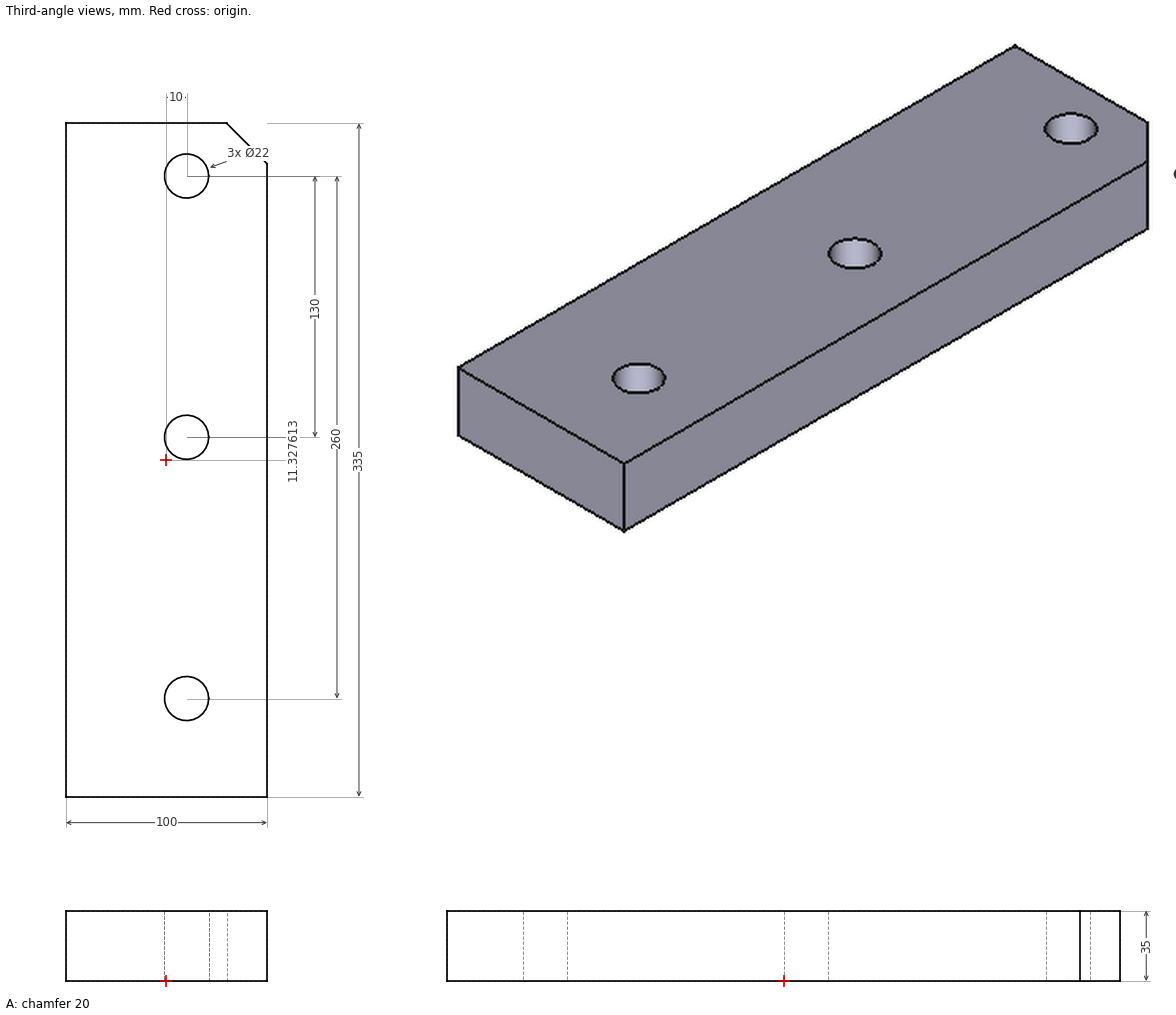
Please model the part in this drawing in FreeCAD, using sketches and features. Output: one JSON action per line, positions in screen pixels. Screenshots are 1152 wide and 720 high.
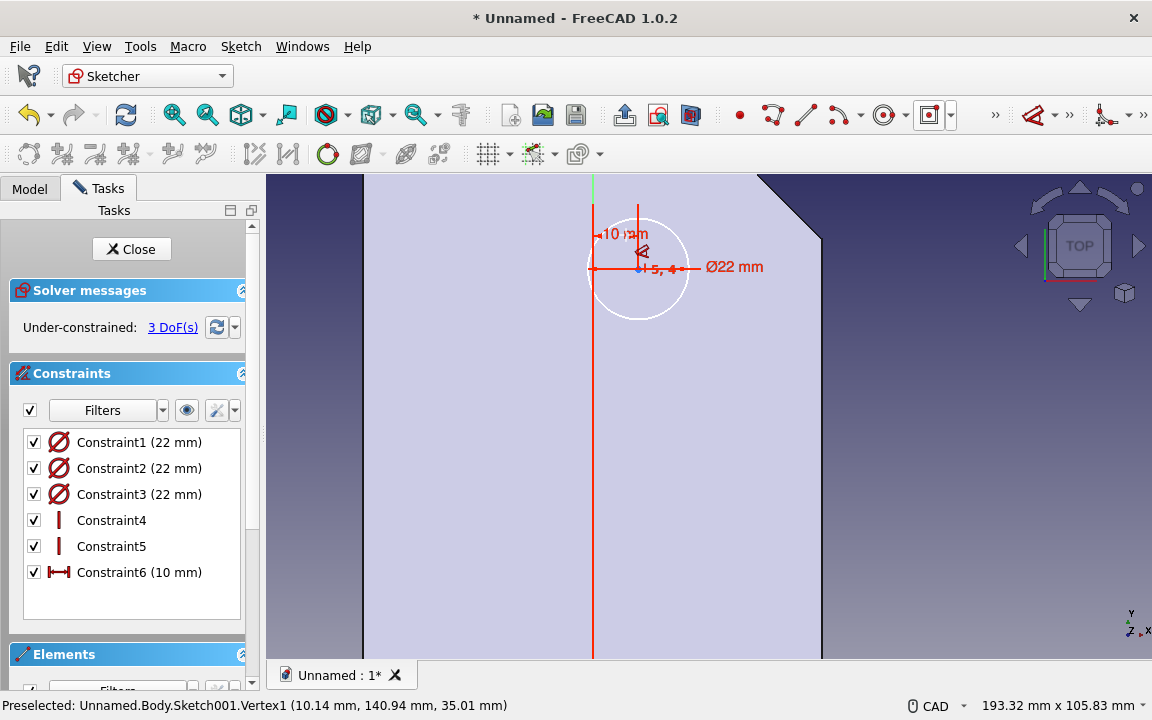
{"action": "scroll", "coordinate": [641, 270], "scroll_direction": "down", "scroll_amount": 7}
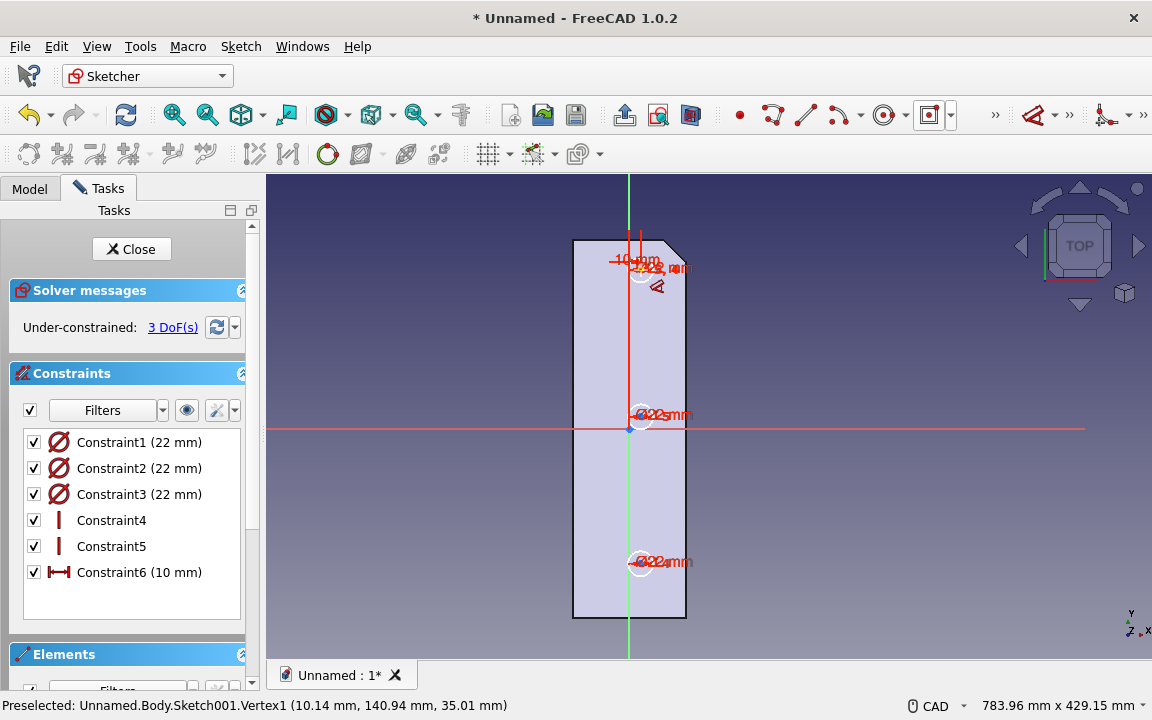
{"action": "left_click", "coordinate": [641, 270]}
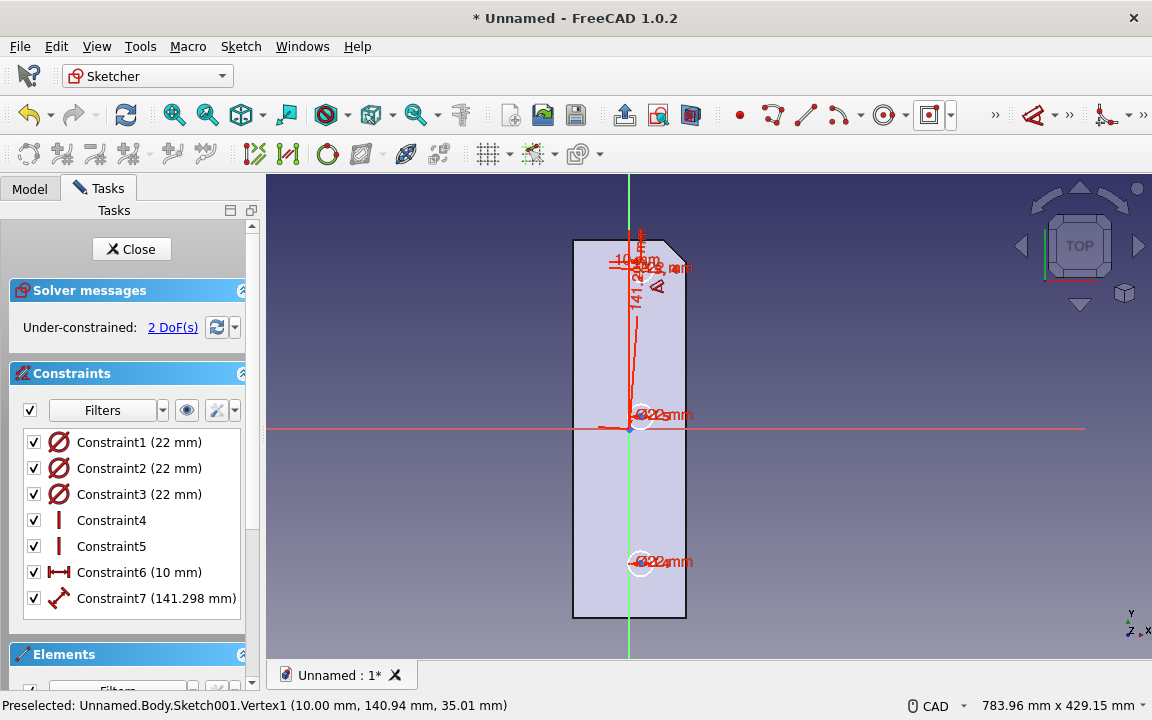
{"action": "left_click", "coordinate": [641, 564]}
{"action": "left_click", "coordinate": [675, 349]}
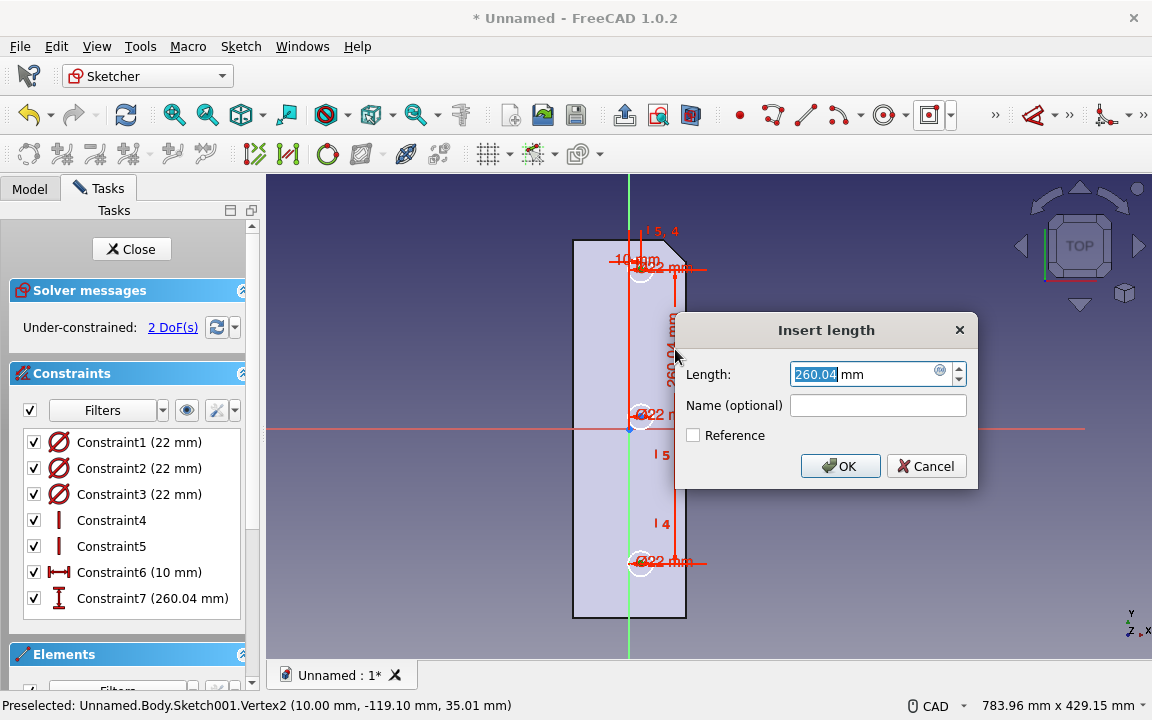
{"action": "type", "text": "260"}
{"action": "key", "text": "Return"}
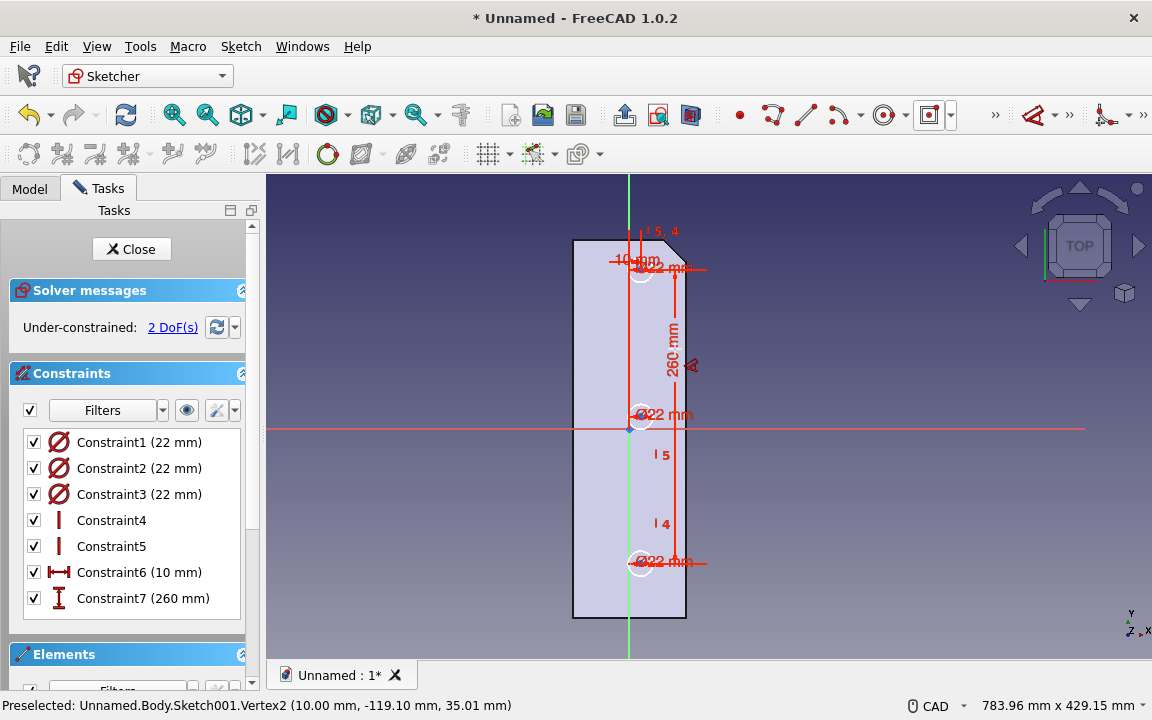
{"action": "left_click", "coordinate": [641, 270]}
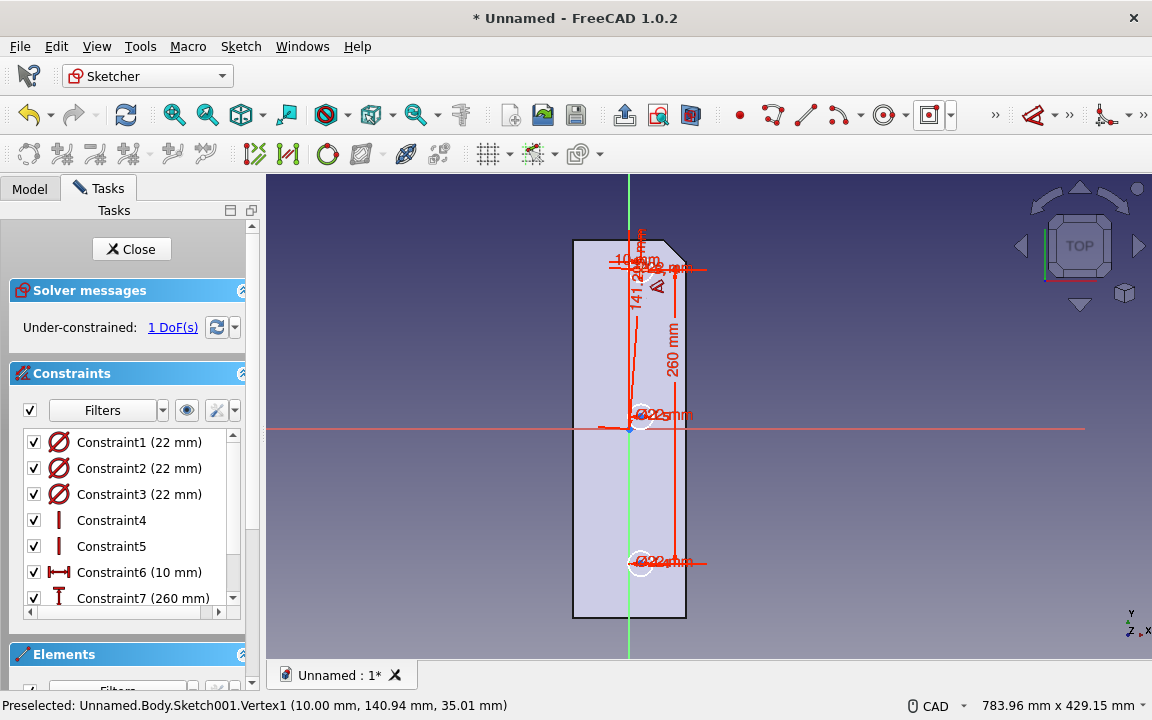
{"action": "left_click", "coordinate": [641, 417]}
{"action": "left_click", "coordinate": [675, 310]}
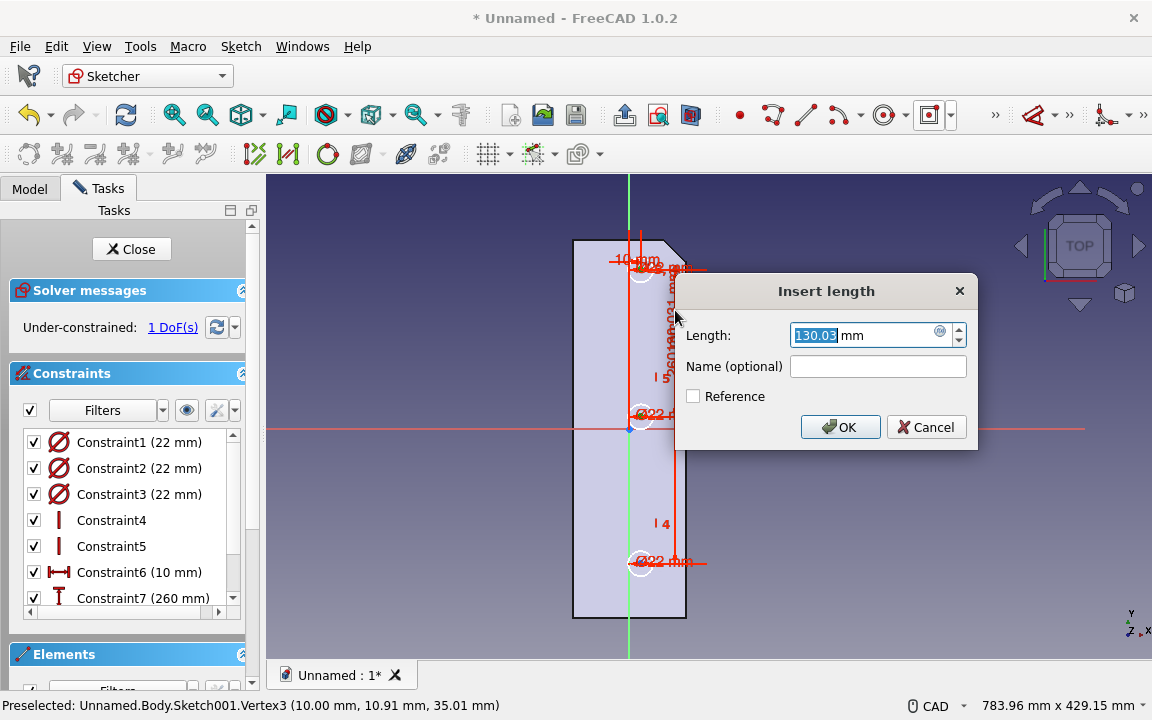
{"action": "type", "text": "130"}
{"action": "key", "text": "Return"}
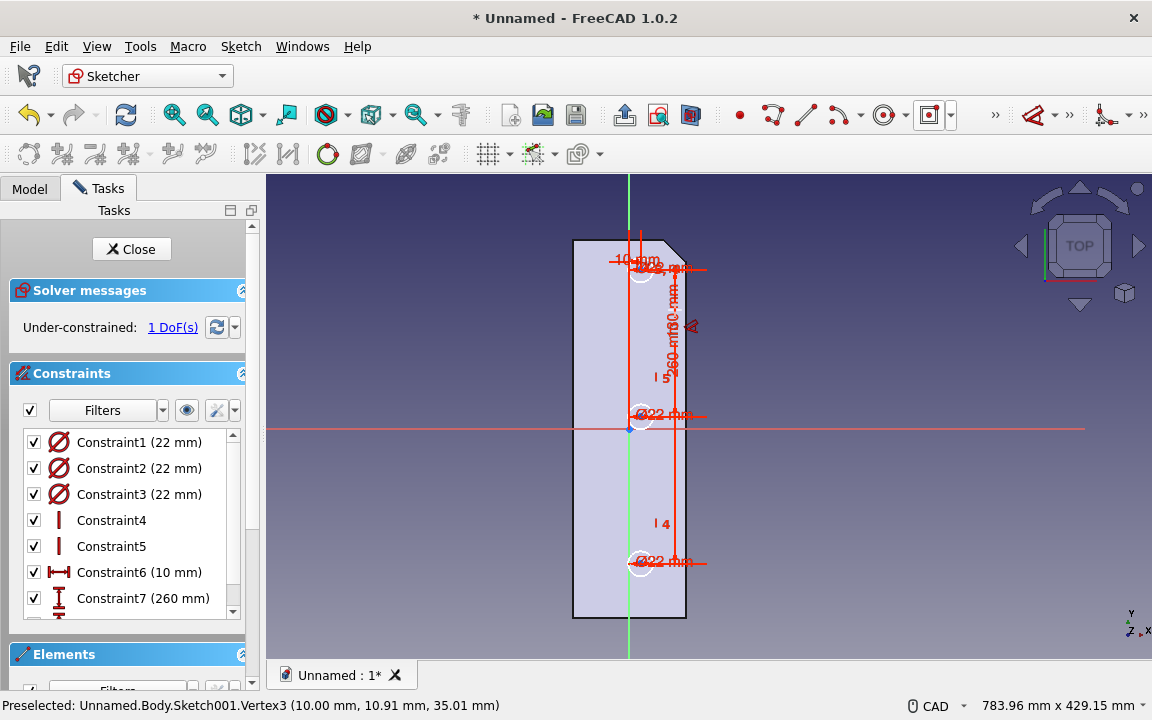
{"action": "scroll", "coordinate": [641, 417], "scroll_direction": "up", "scroll_amount": 6}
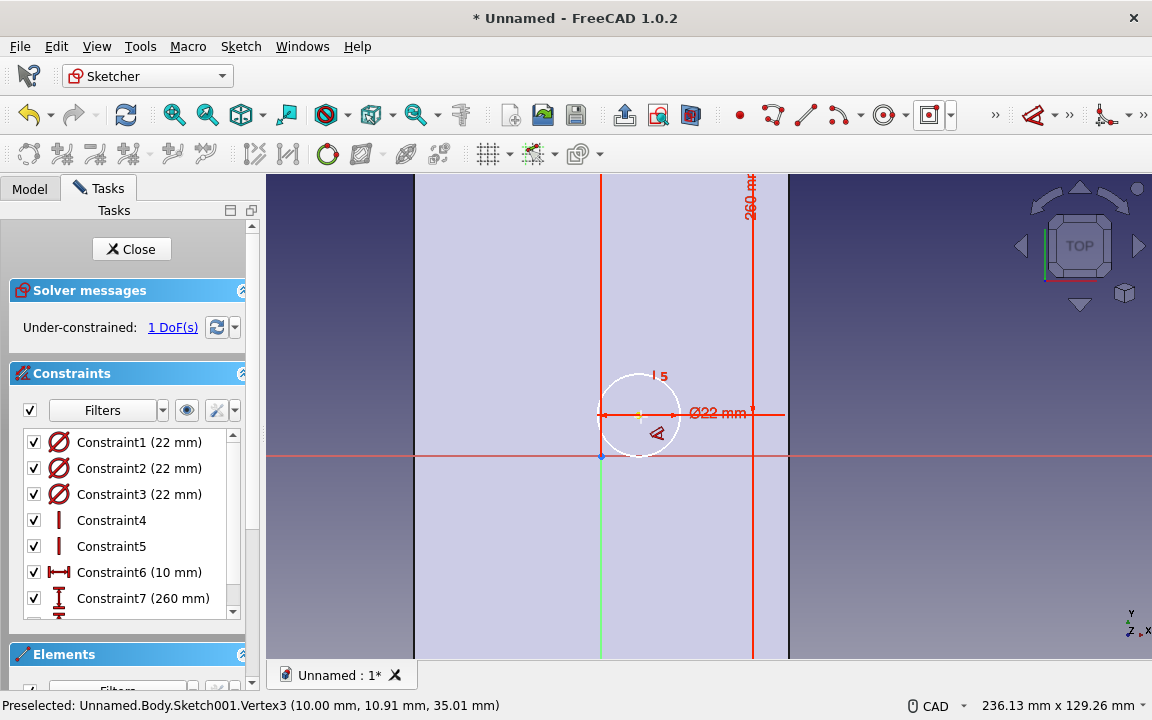
{"action": "left_click", "coordinate": [639, 415]}
{"action": "left_click", "coordinate": [567, 436]}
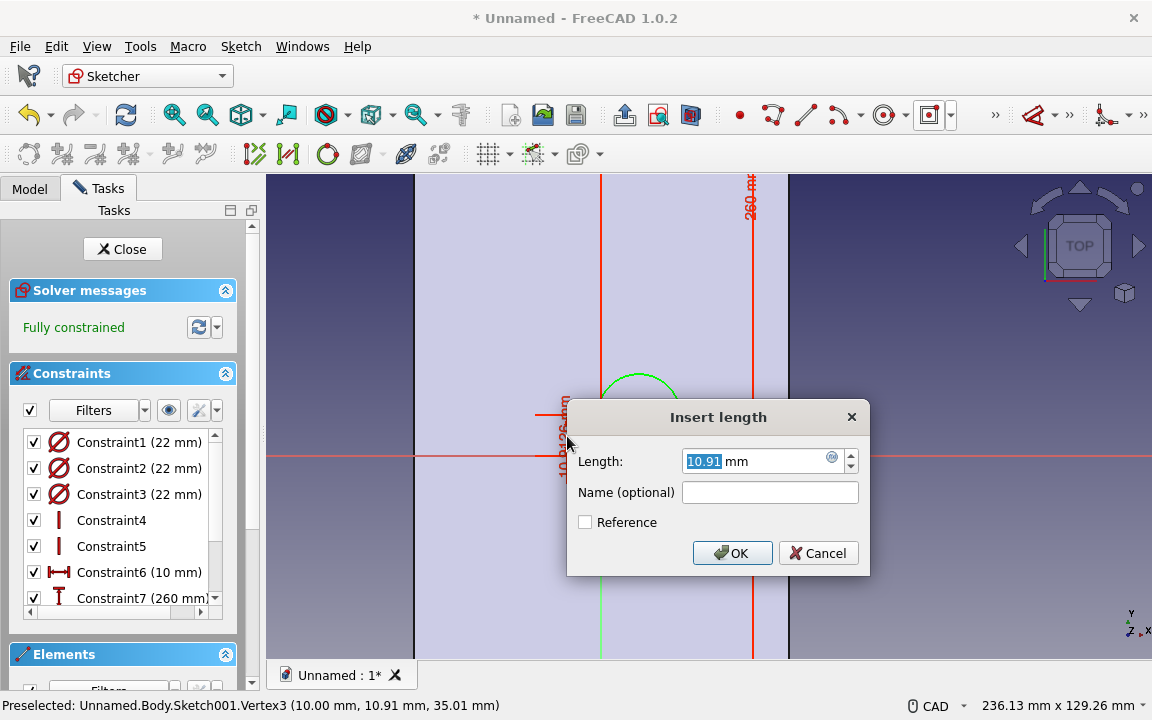
{"action": "type", "text": "11.327613"}
{"action": "key", "text": "Return"}
{"action": "key", "text": "Escape"}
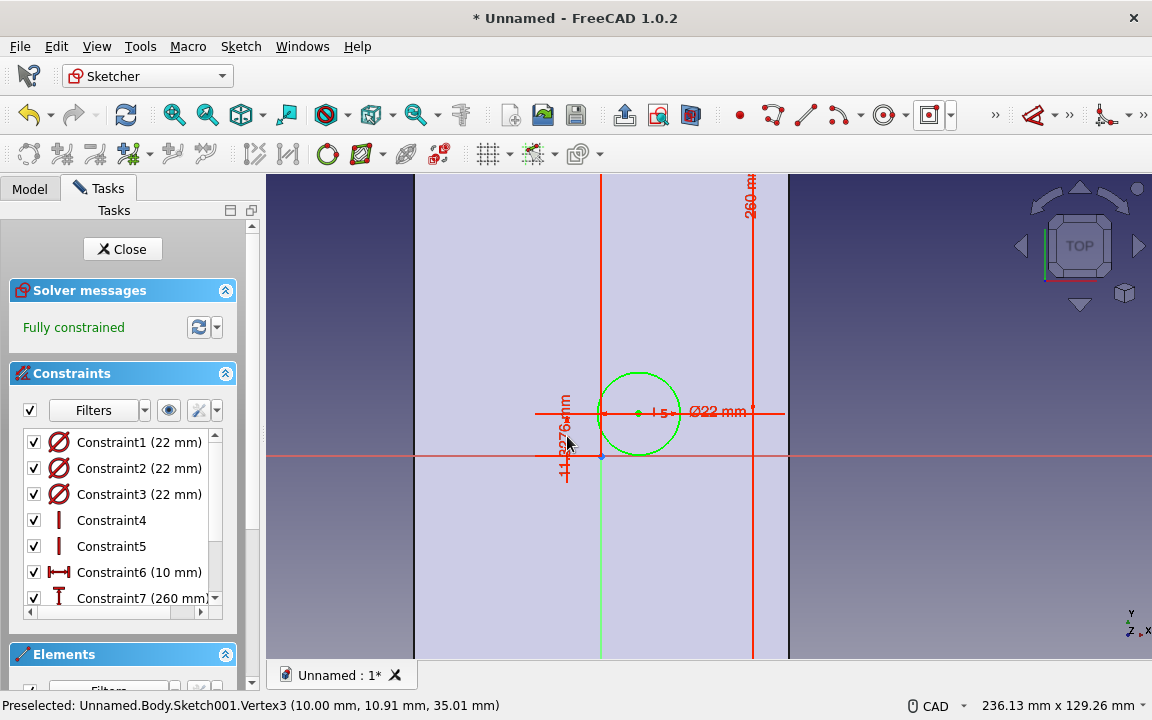
{"action": "left_click", "coordinate": [123, 249]}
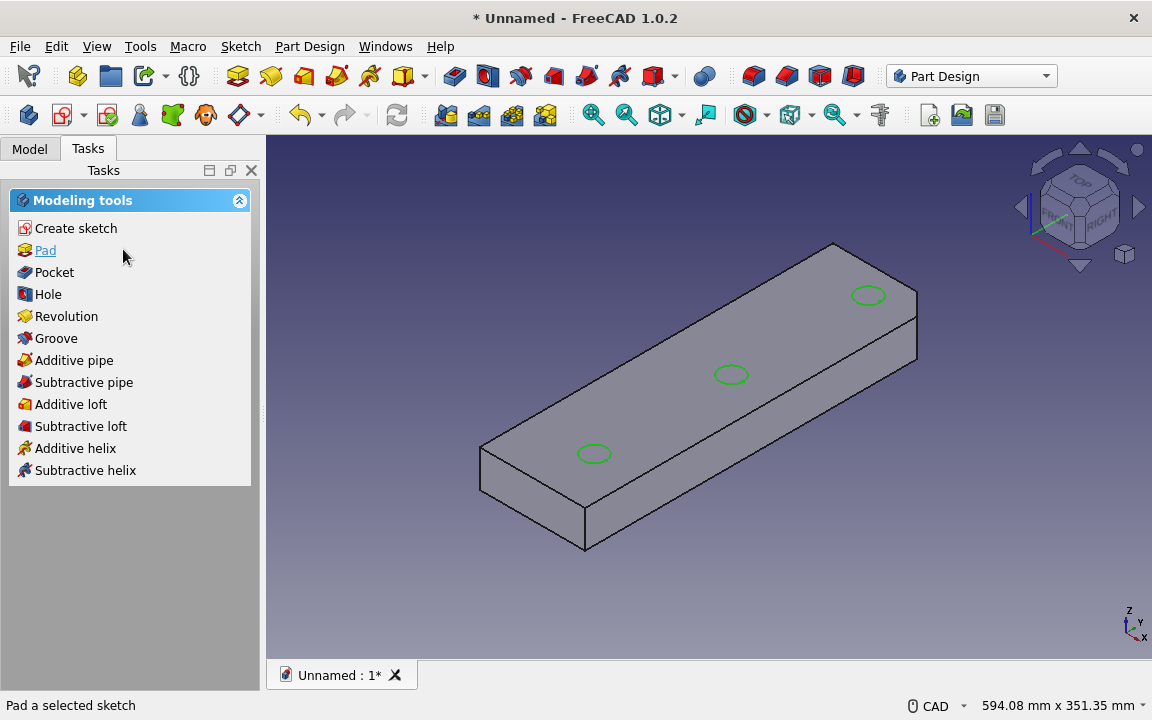
{"action": "left_click", "coordinate": [455, 76]}